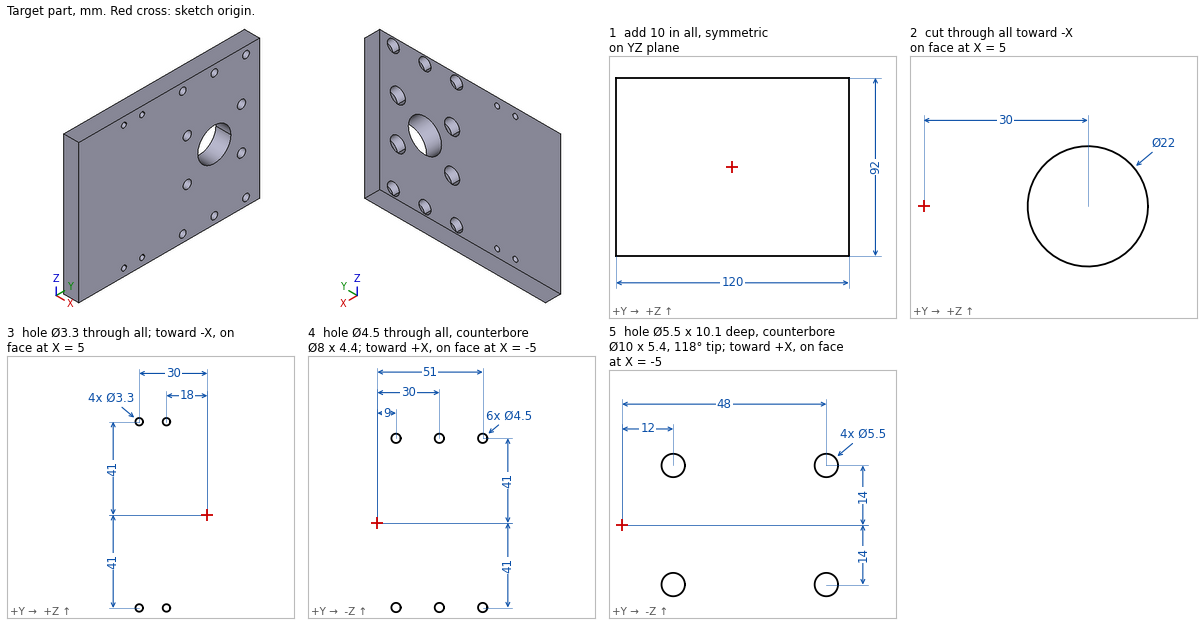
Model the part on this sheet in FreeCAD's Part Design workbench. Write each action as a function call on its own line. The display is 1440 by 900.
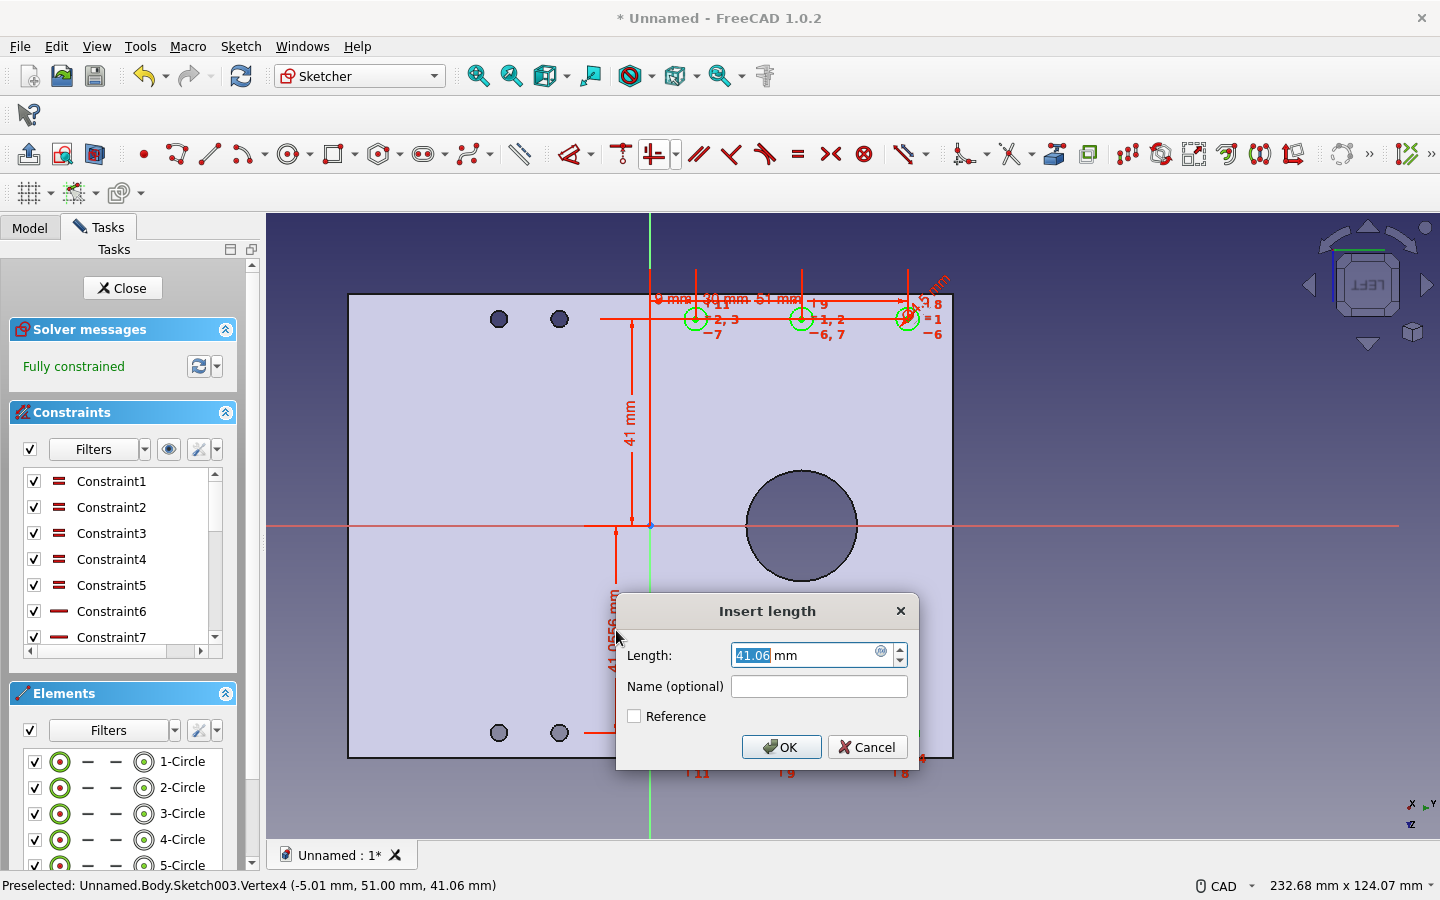
text(41)
key(Return)
key(Escape)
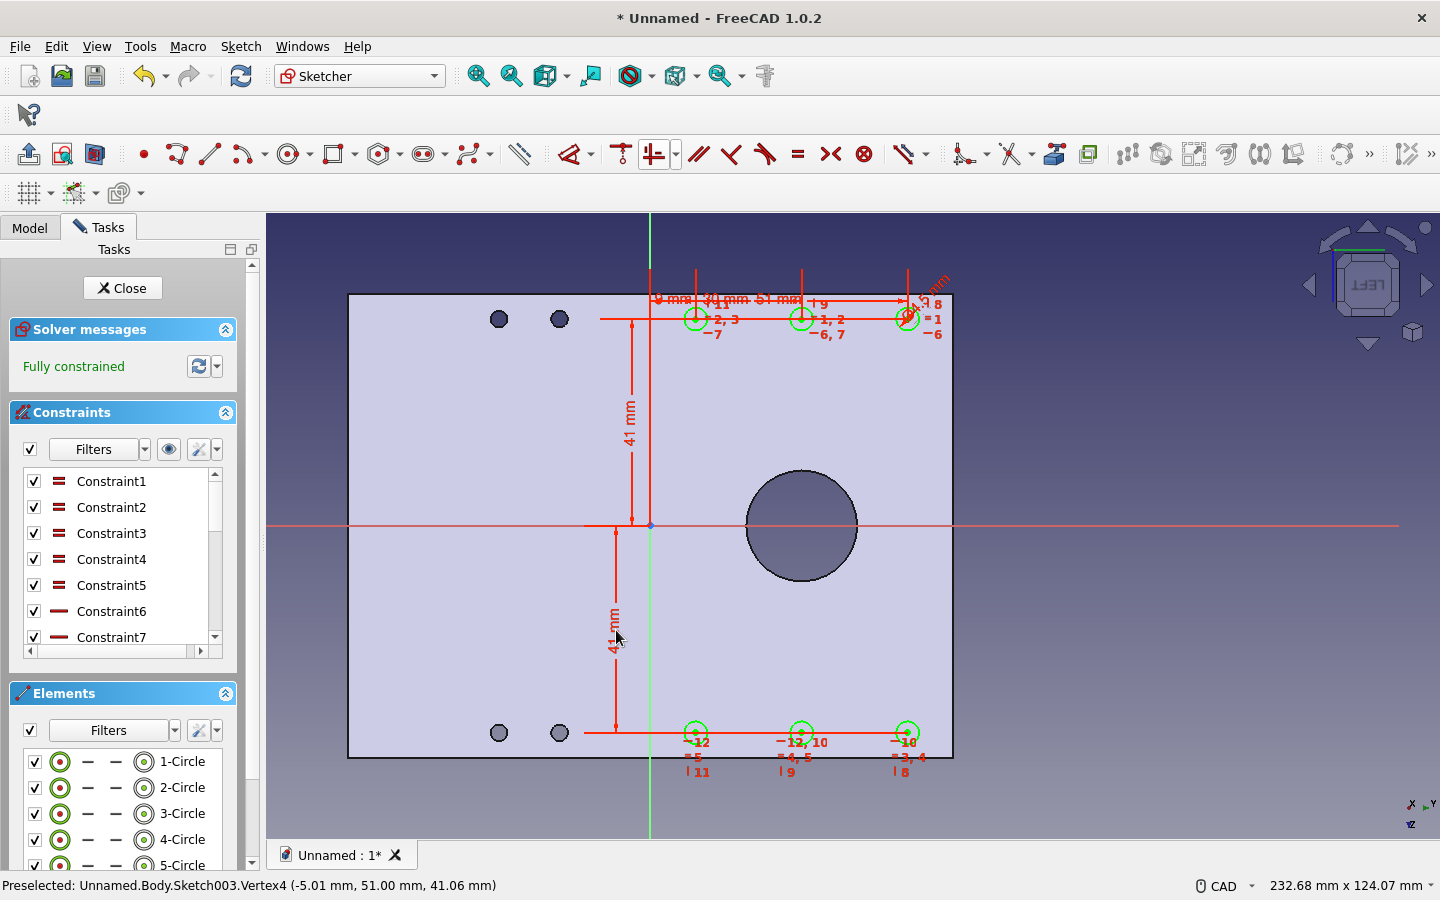
click(123, 288)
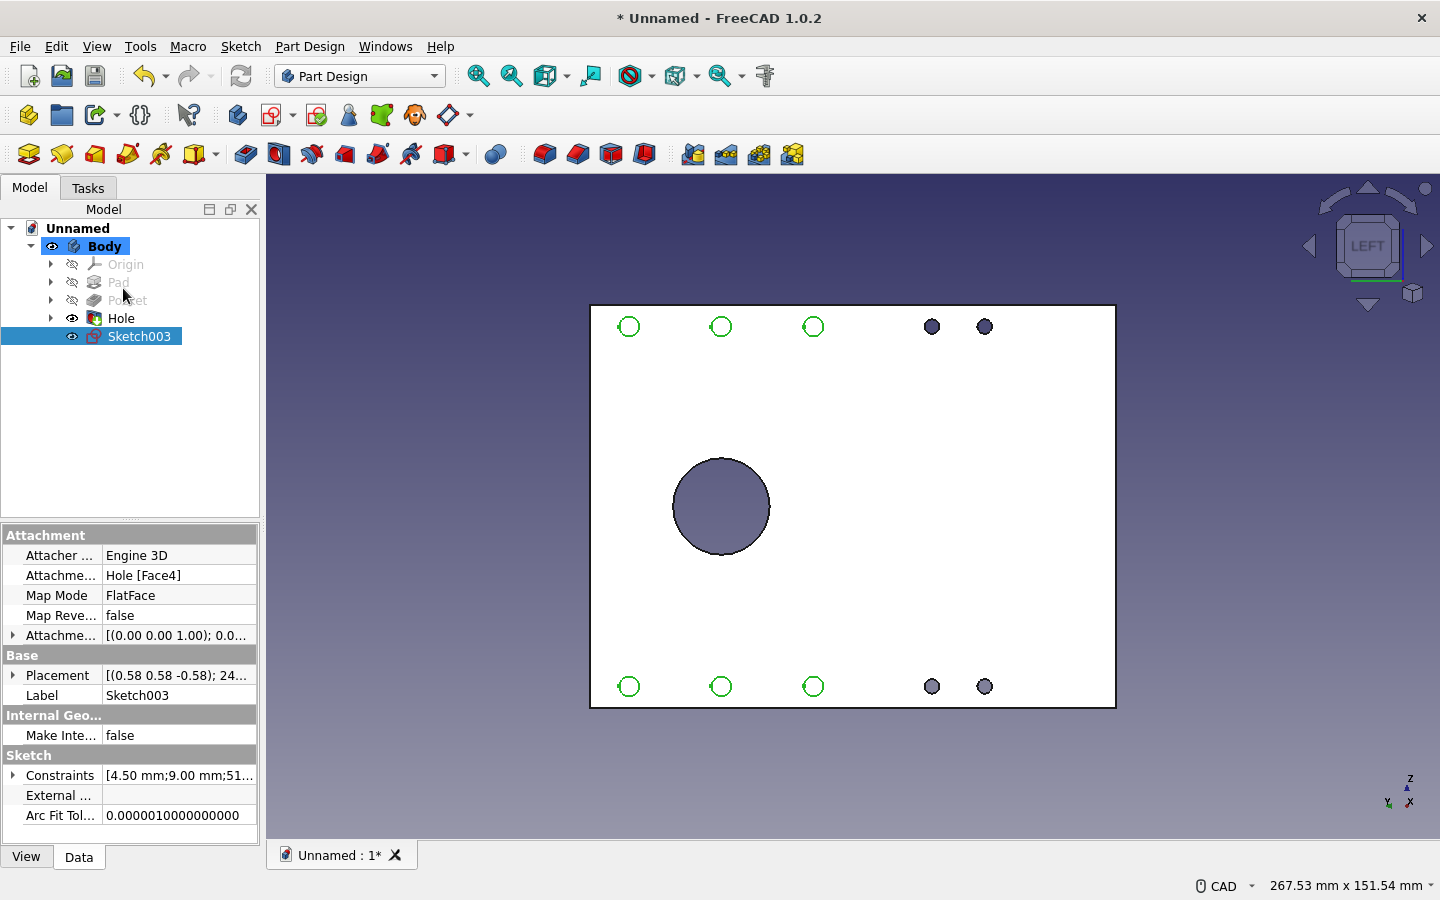
click(279, 154)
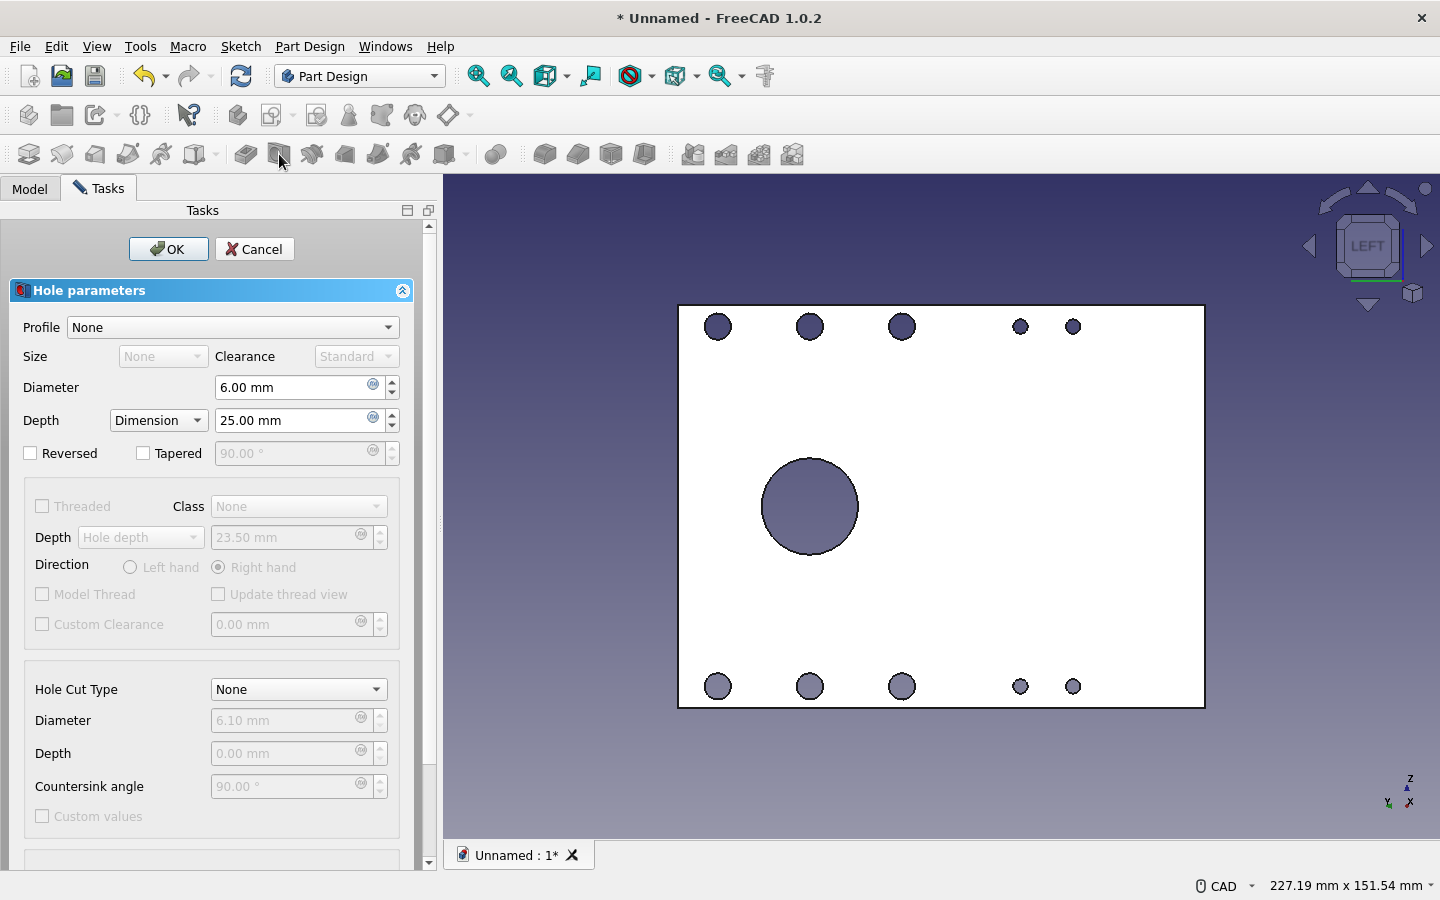
triple_click(300, 388)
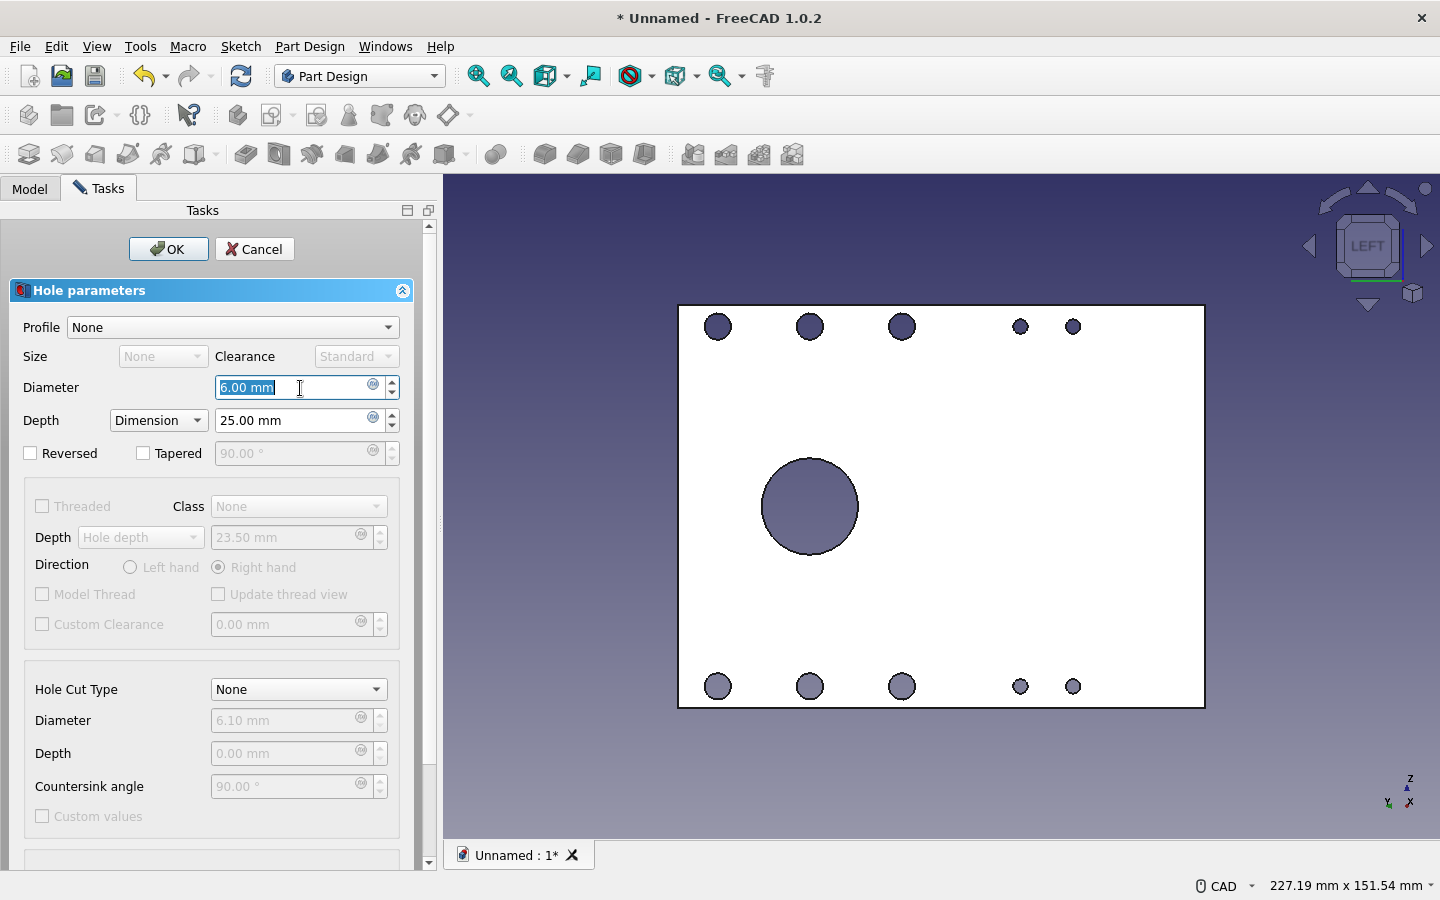
text(4.5)
key(Tab)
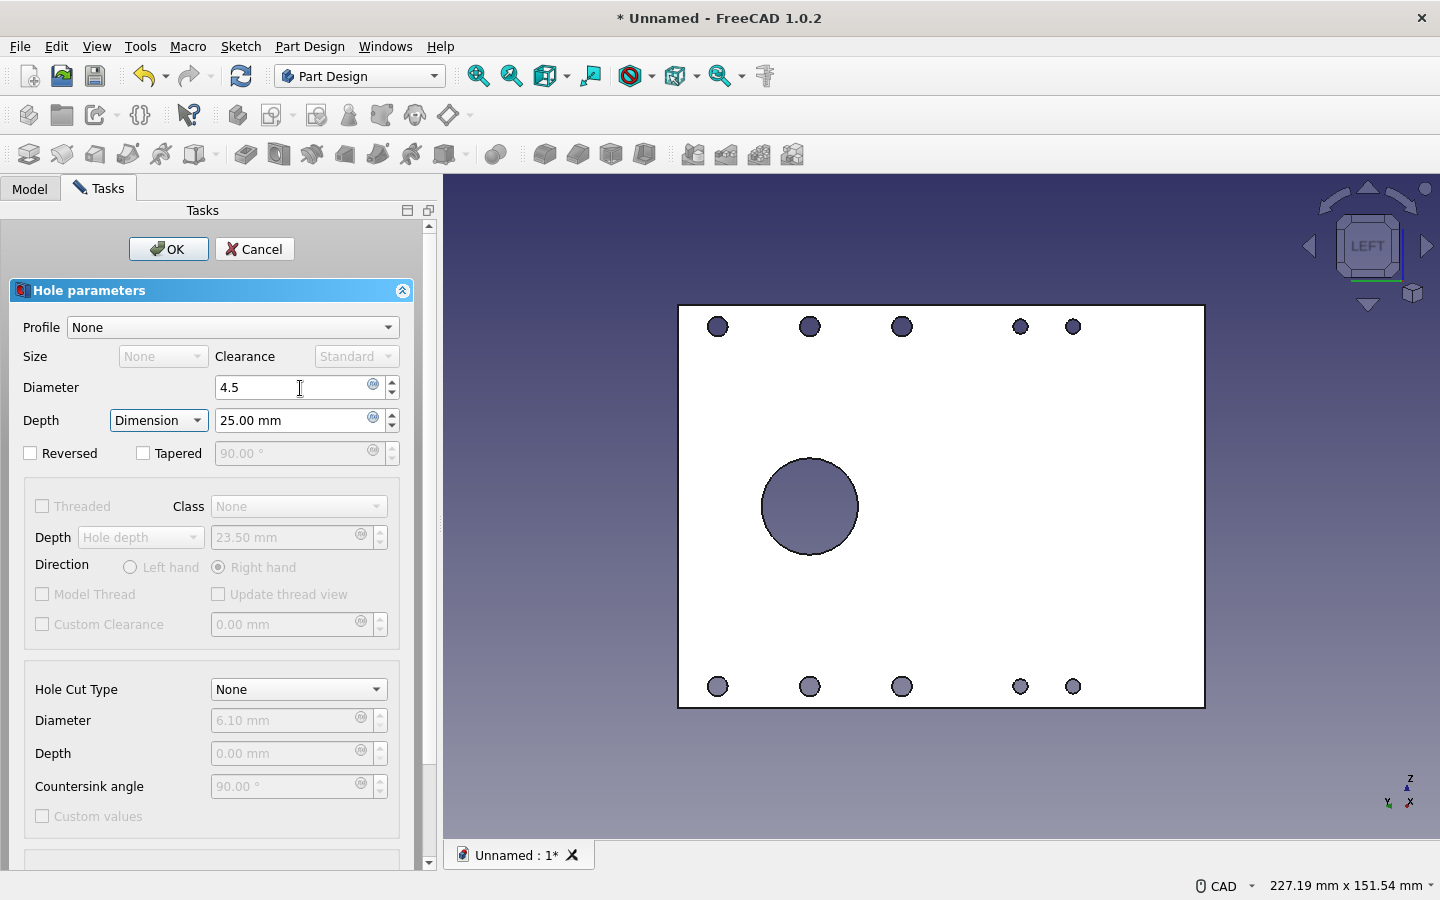
click(160, 420)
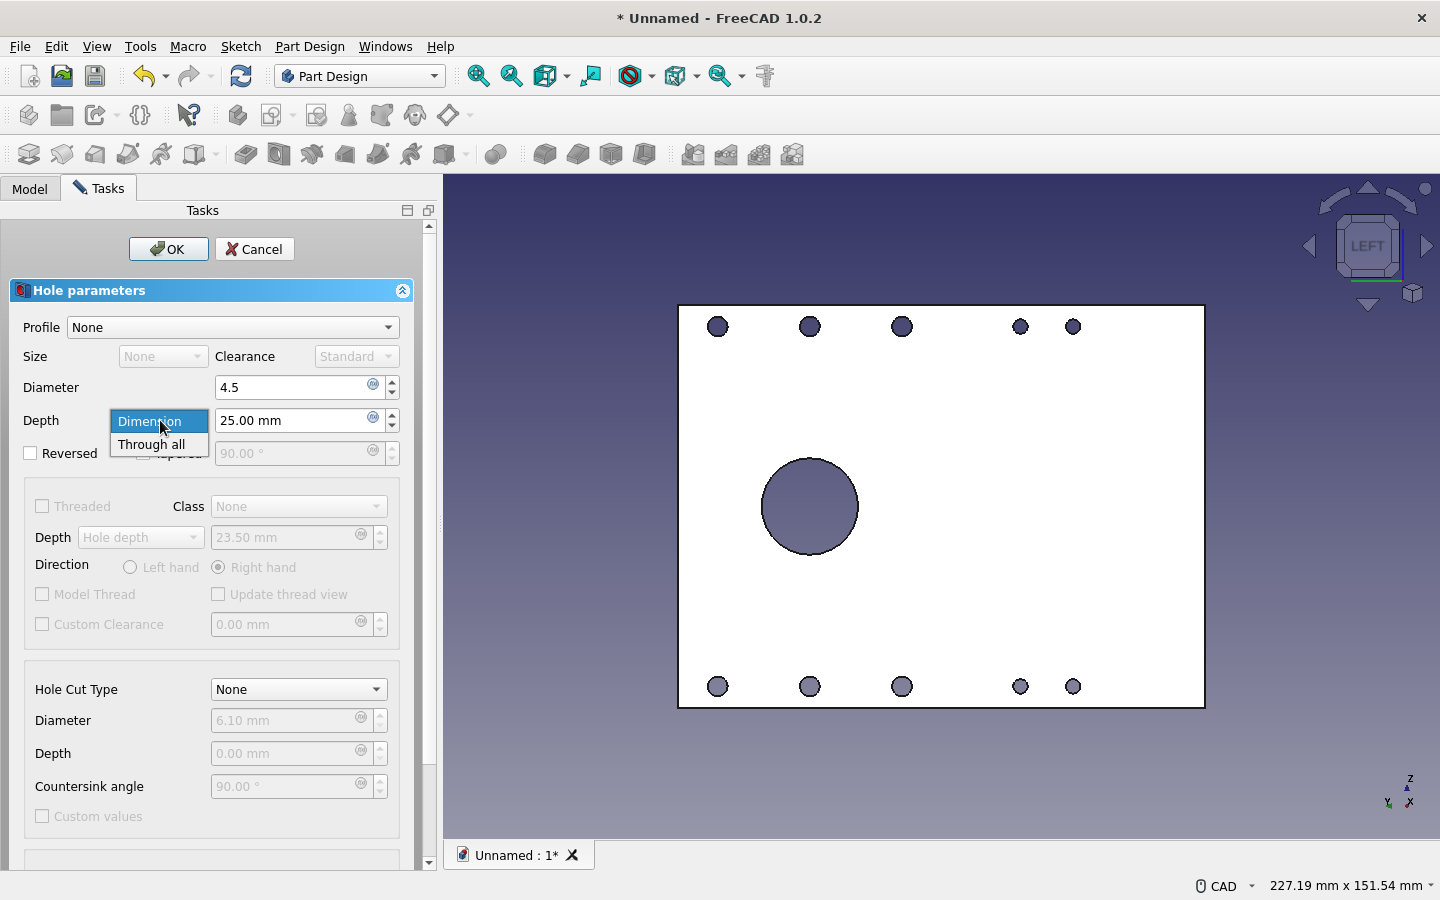
click(158, 444)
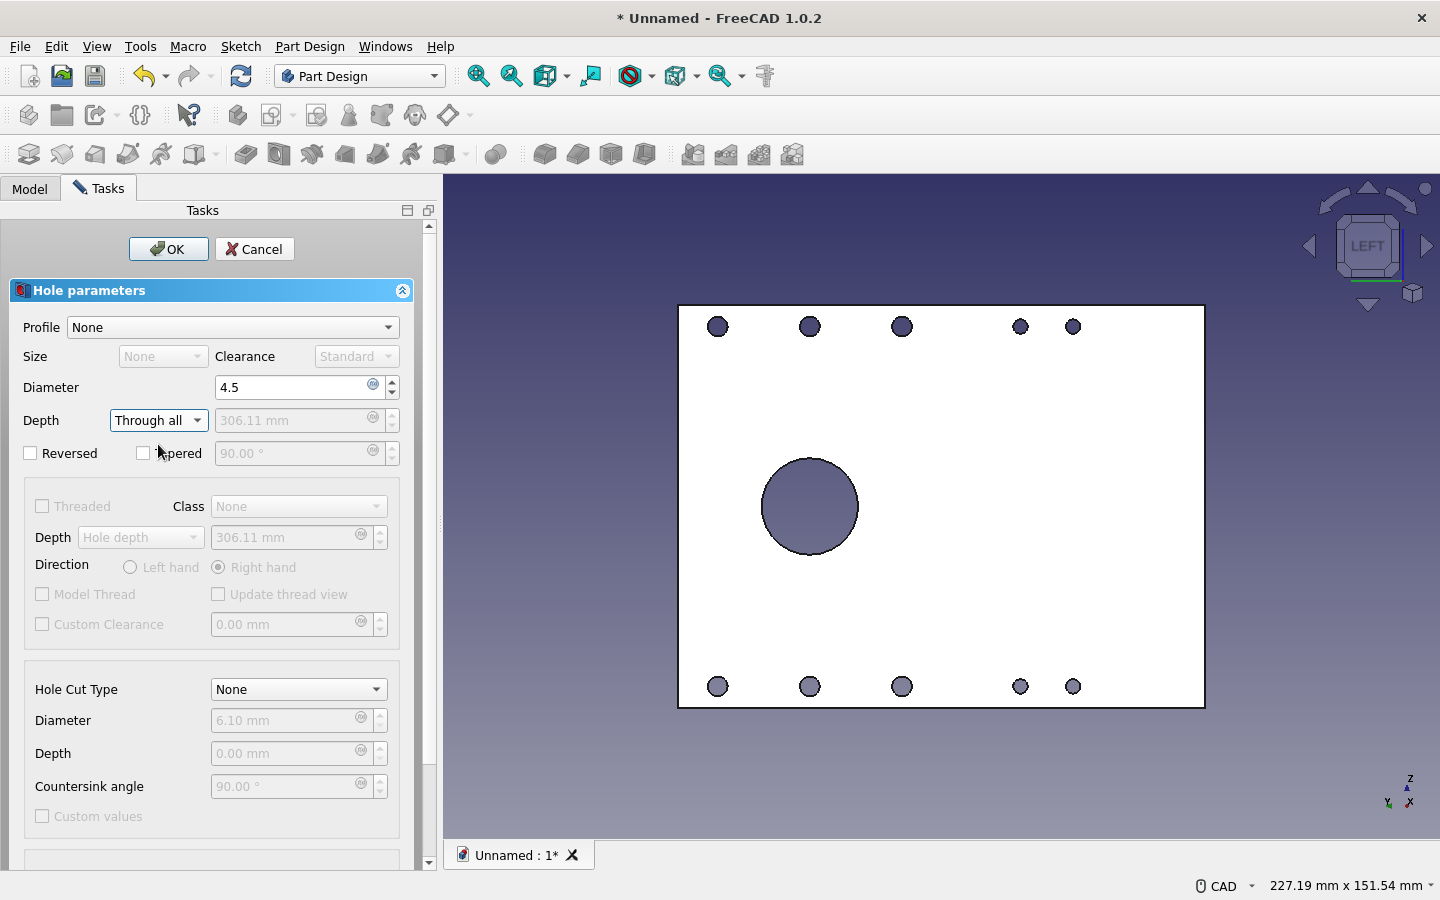
click(300, 690)